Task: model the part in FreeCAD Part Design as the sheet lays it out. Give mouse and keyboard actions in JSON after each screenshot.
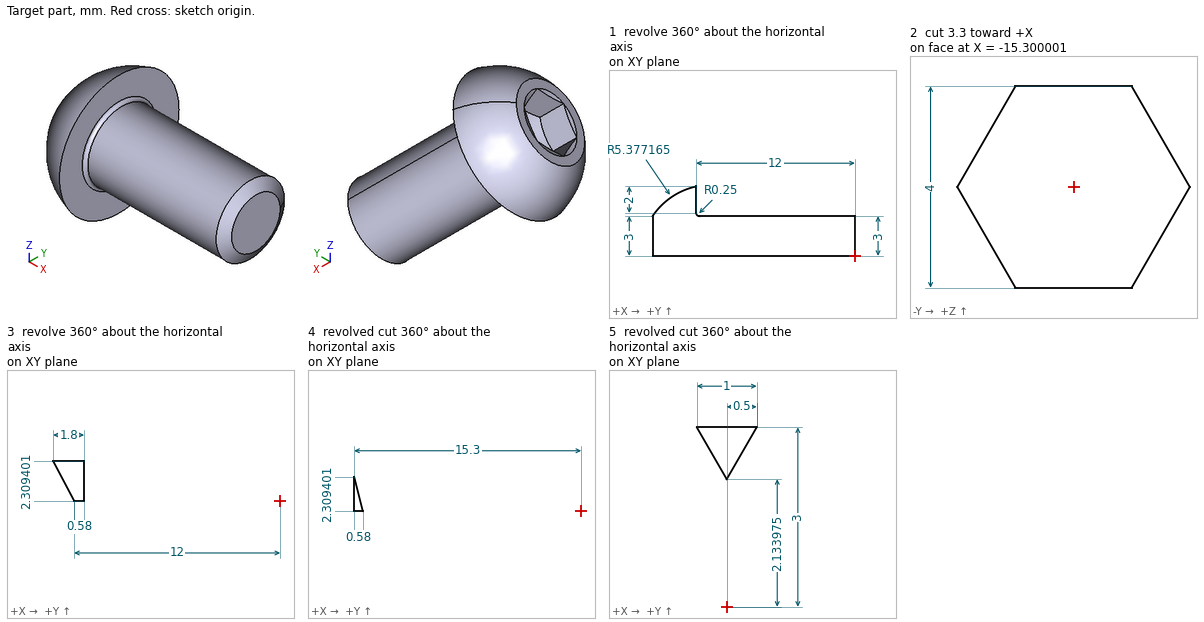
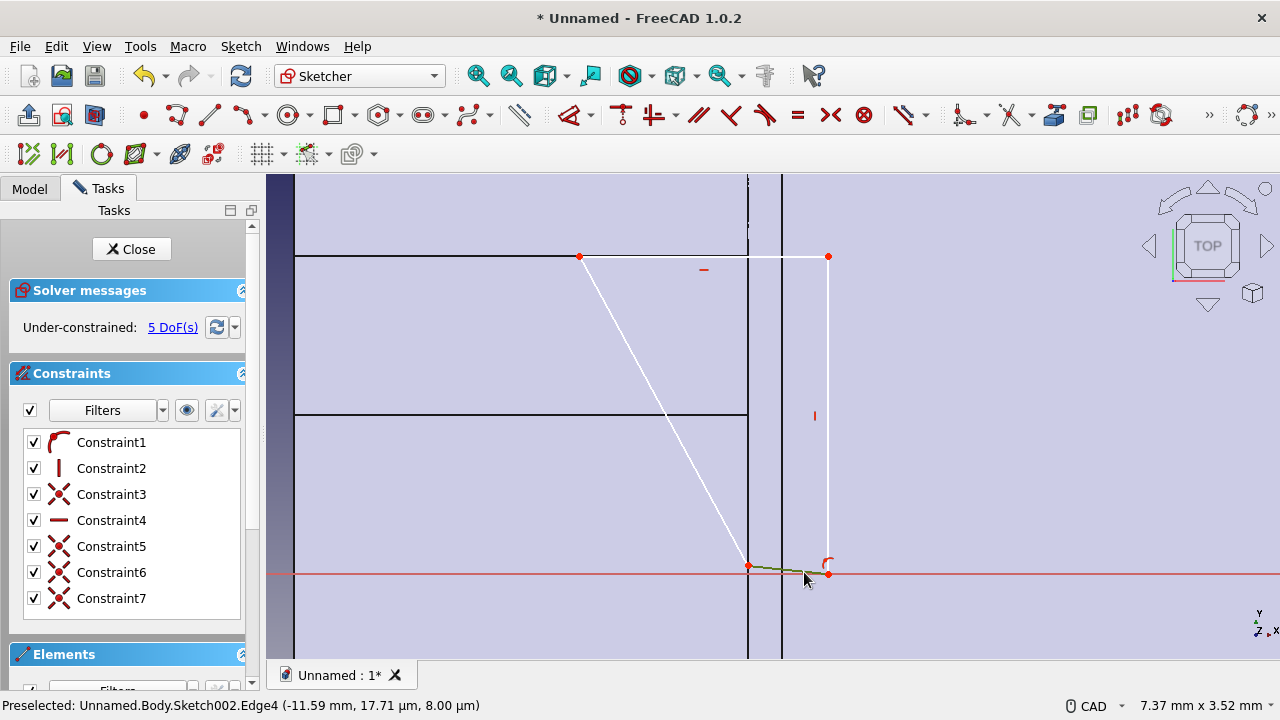
{"action": "key", "text": "h"}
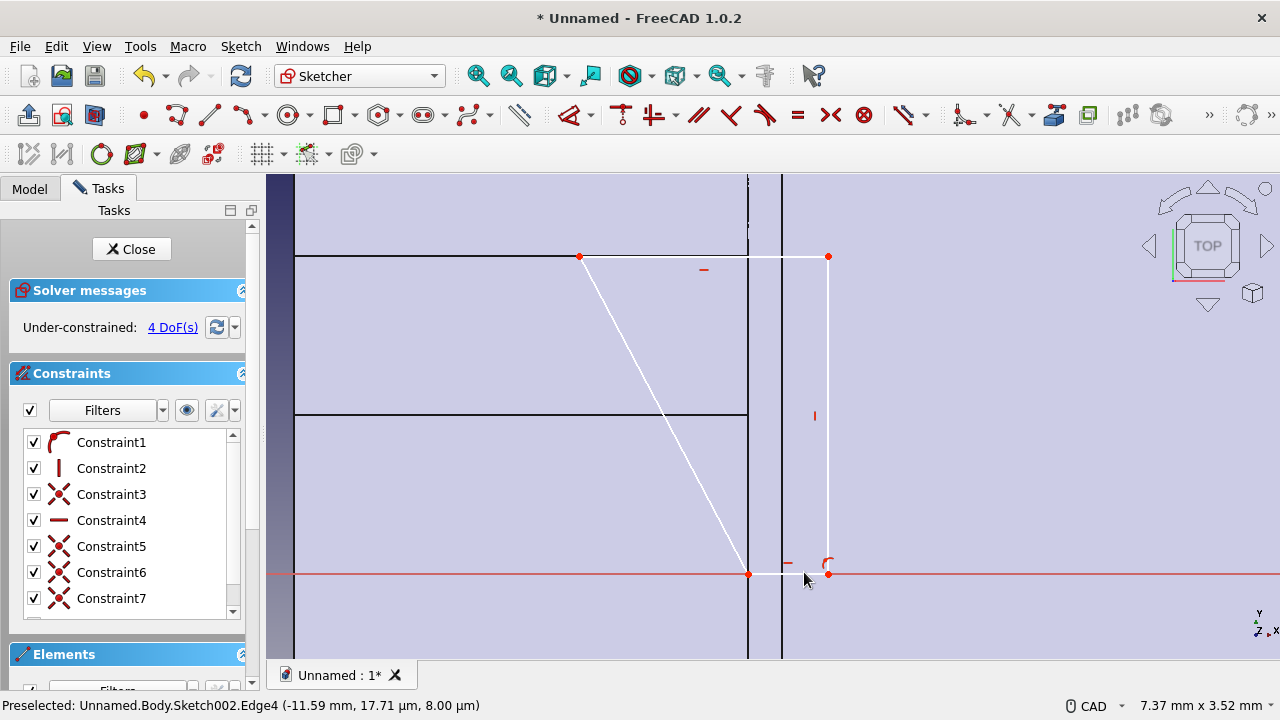
{"action": "left_click", "coordinate": [568, 116]}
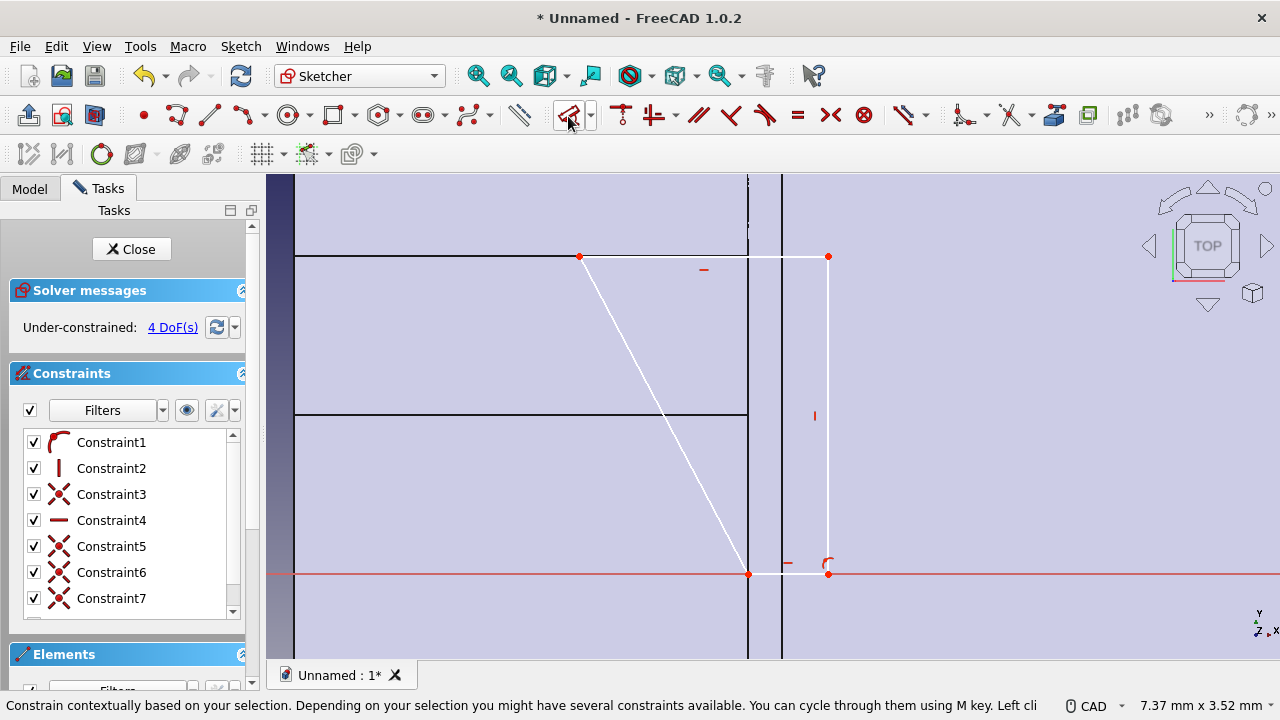
{"action": "left_click", "coordinate": [754, 257]}
{"action": "left_click", "coordinate": [704, 223]}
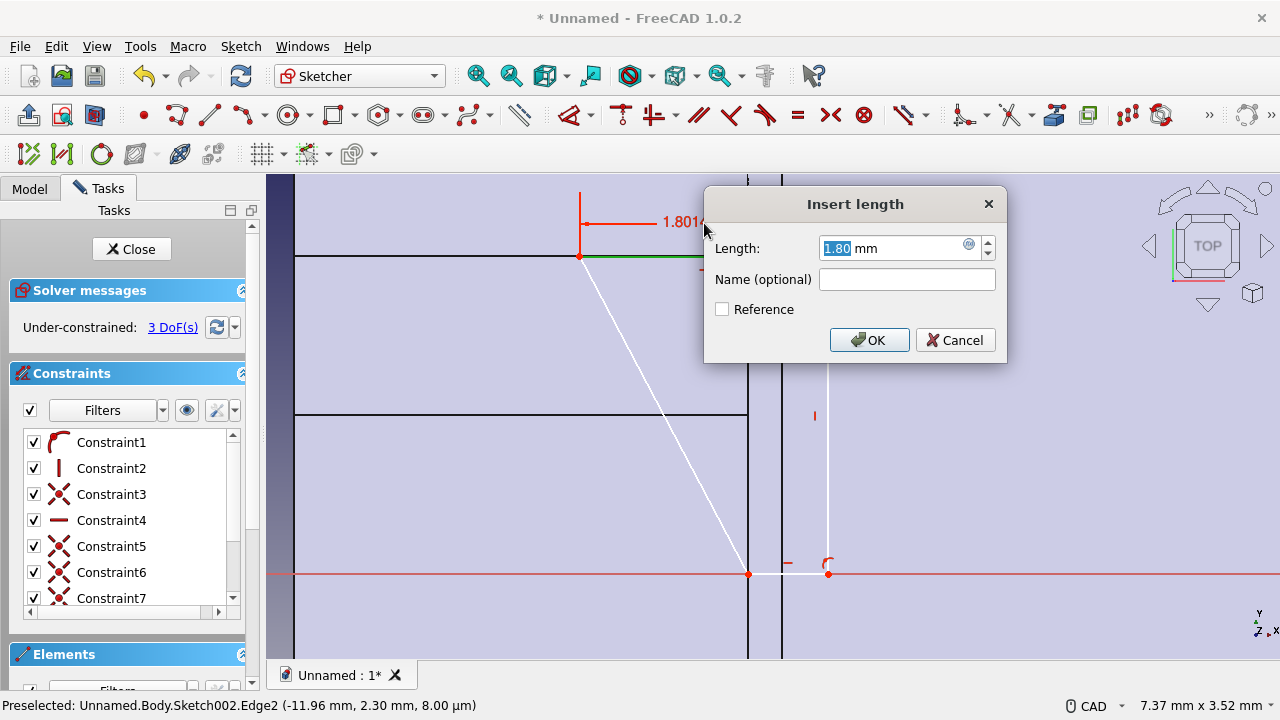
{"action": "type", "text": "1.8"}
{"action": "key", "text": "Return"}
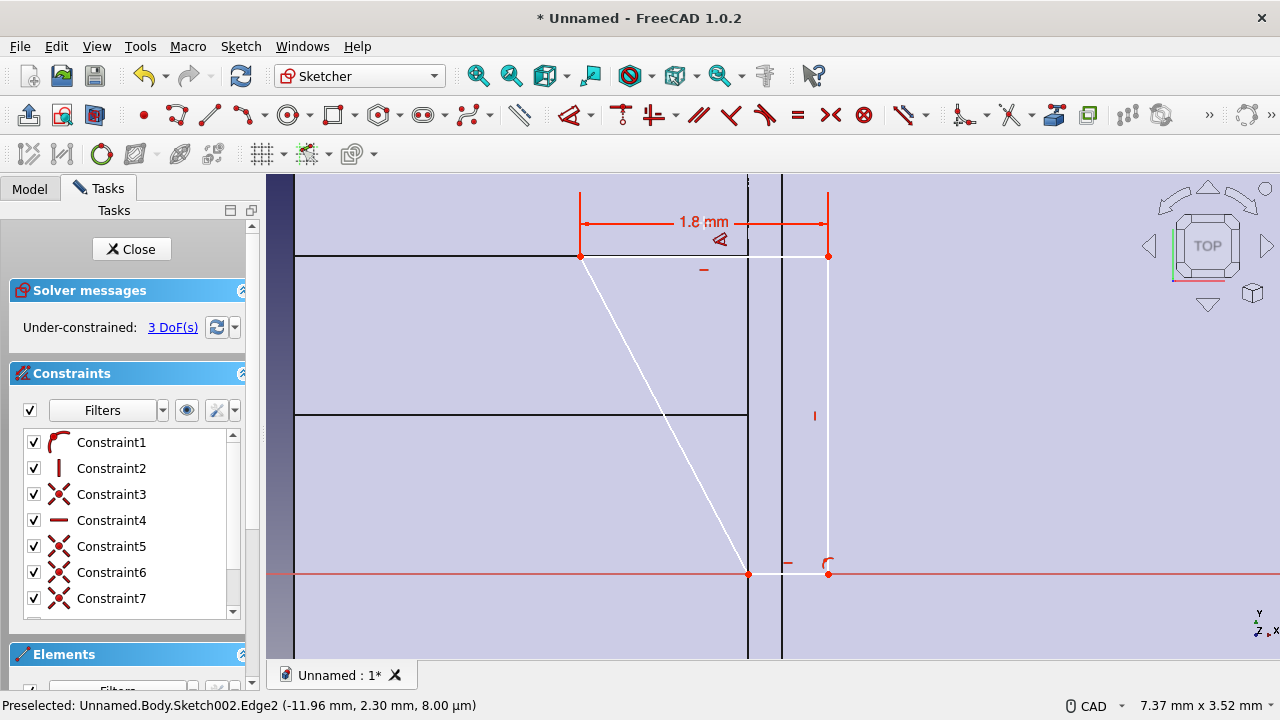
{"action": "left_click", "coordinate": [748, 574]}
{"action": "left_click", "coordinate": [932, 608]}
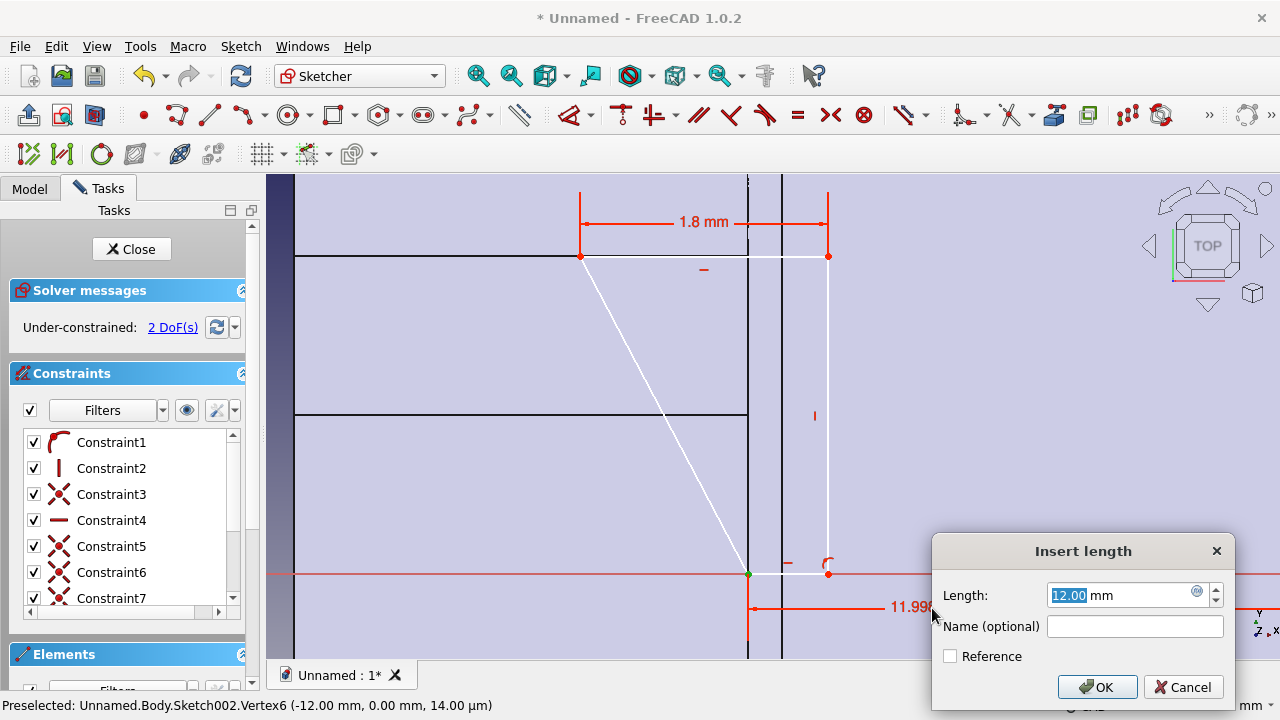
{"action": "type", "text": "12"}
{"action": "key", "text": "Return"}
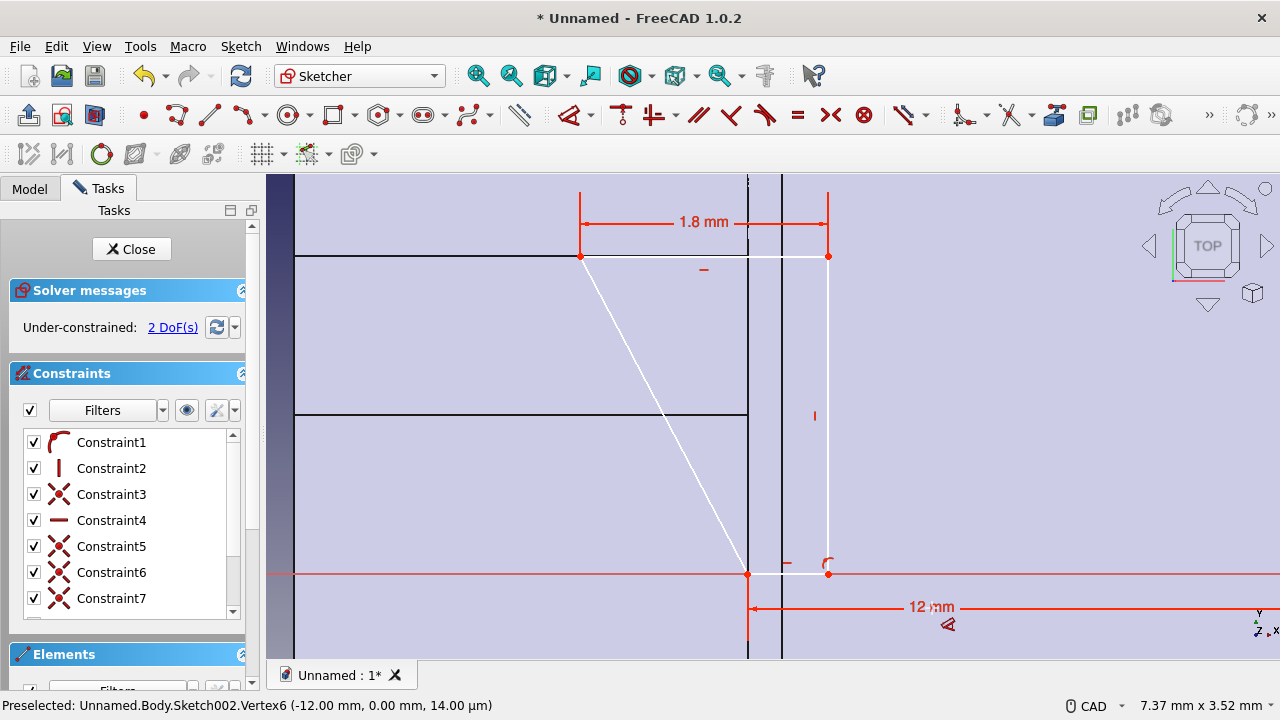
{"action": "left_click", "coordinate": [772, 574]}
{"action": "left_click", "coordinate": [788, 608]}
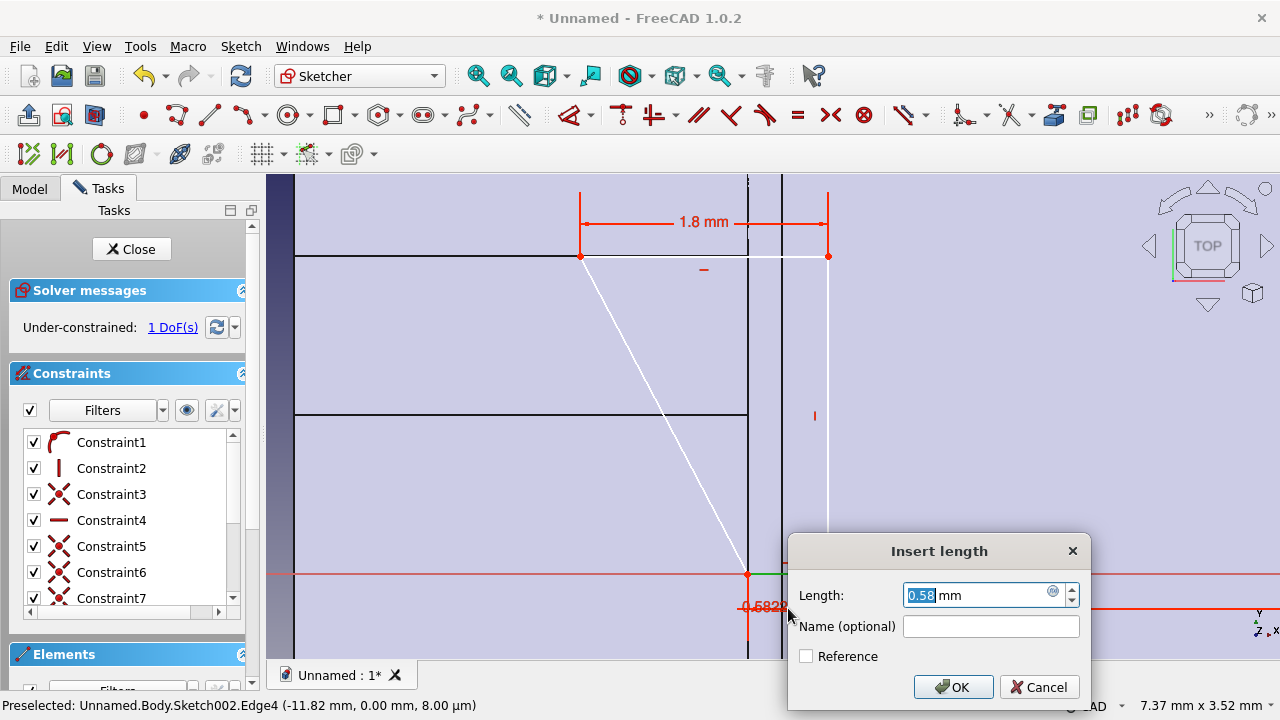
{"action": "type", "text": "0.58"}
{"action": "key", "text": "Return"}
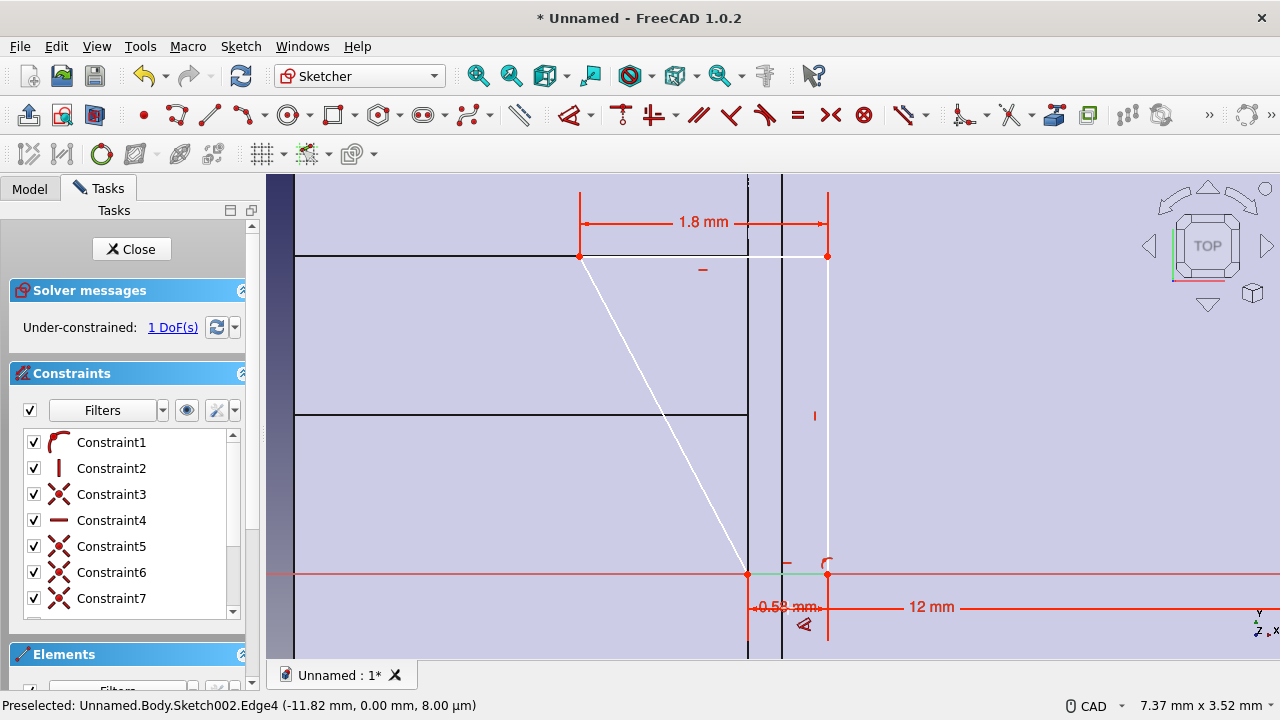
{"action": "left_click", "coordinate": [828, 479]}
{"action": "left_click", "coordinate": [862, 416]}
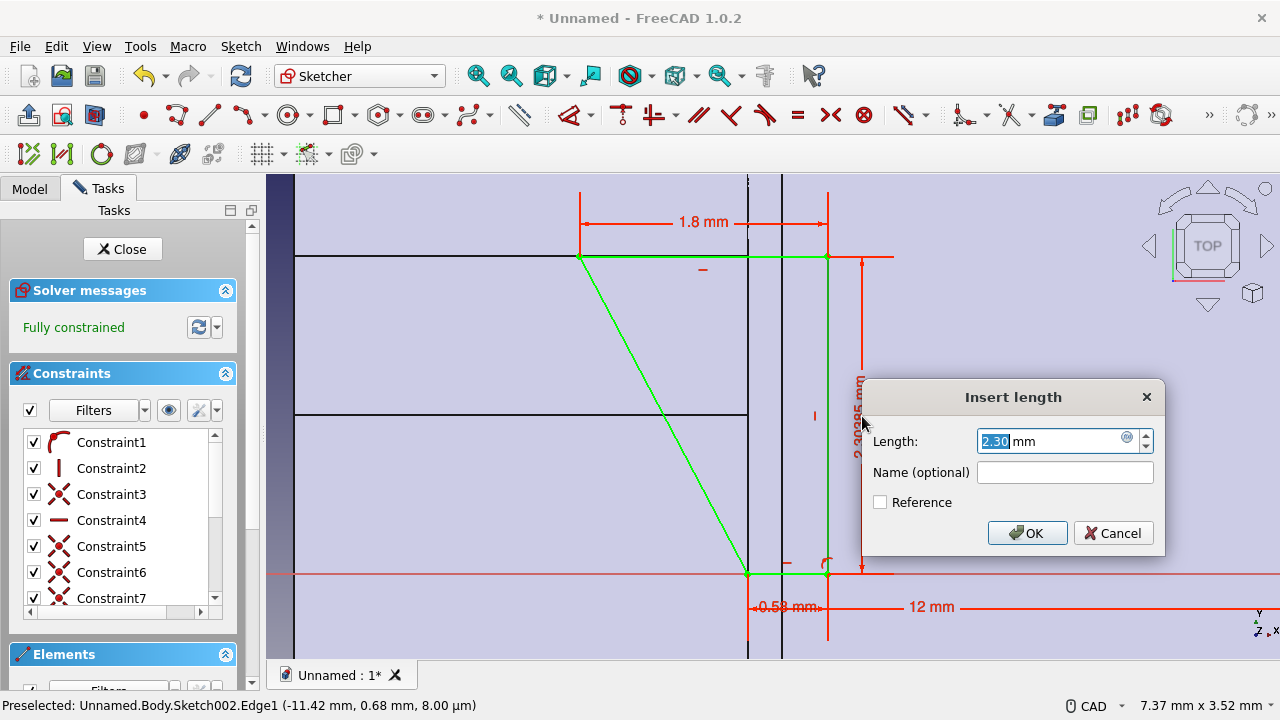
{"action": "type", "text": "2.309401"}
{"action": "key", "text": "Return"}
{"action": "key", "text": "Escape"}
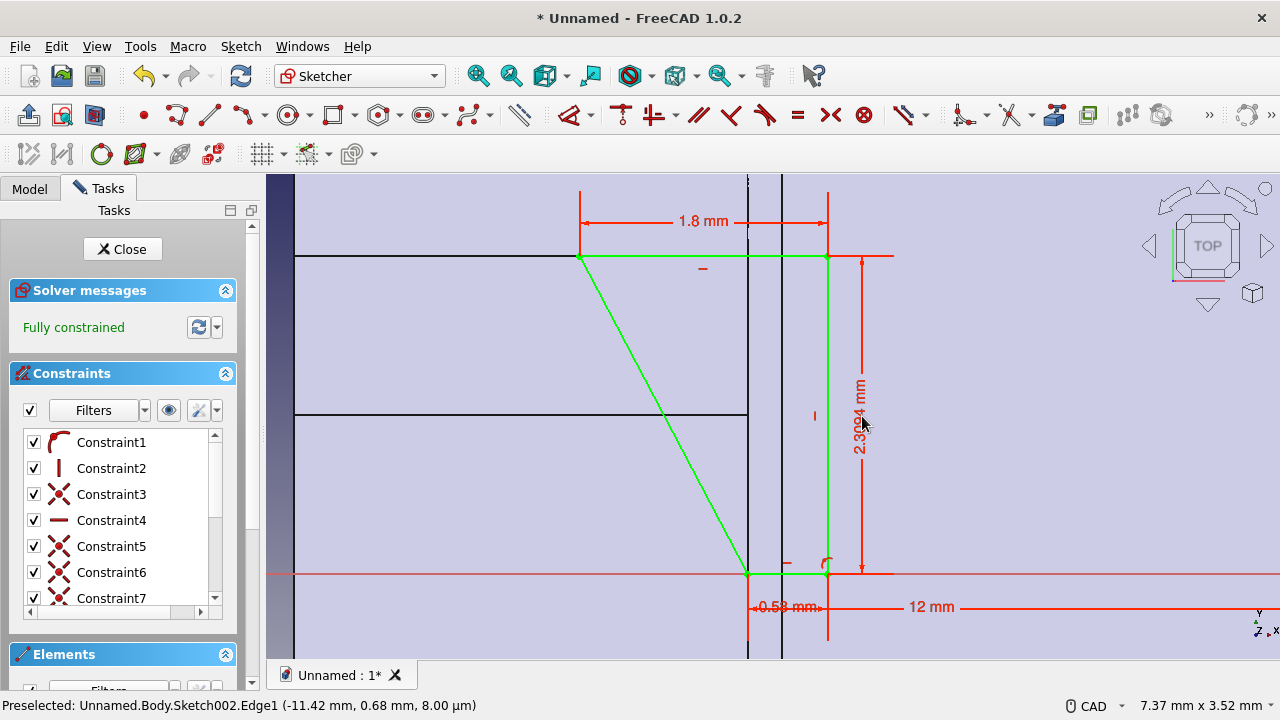
{"action": "left_click", "coordinate": [123, 249]}